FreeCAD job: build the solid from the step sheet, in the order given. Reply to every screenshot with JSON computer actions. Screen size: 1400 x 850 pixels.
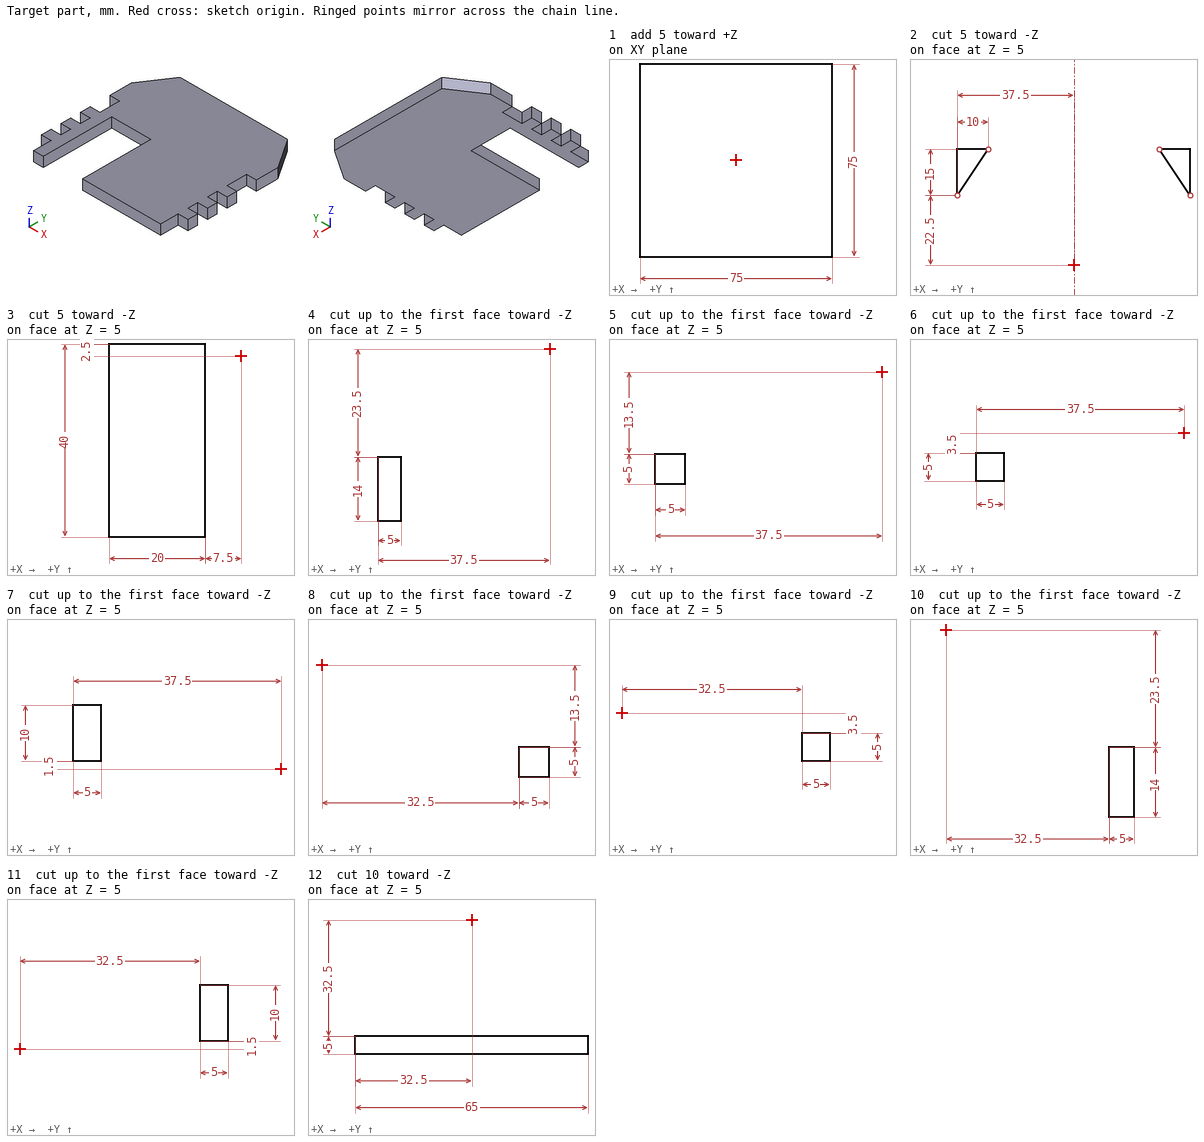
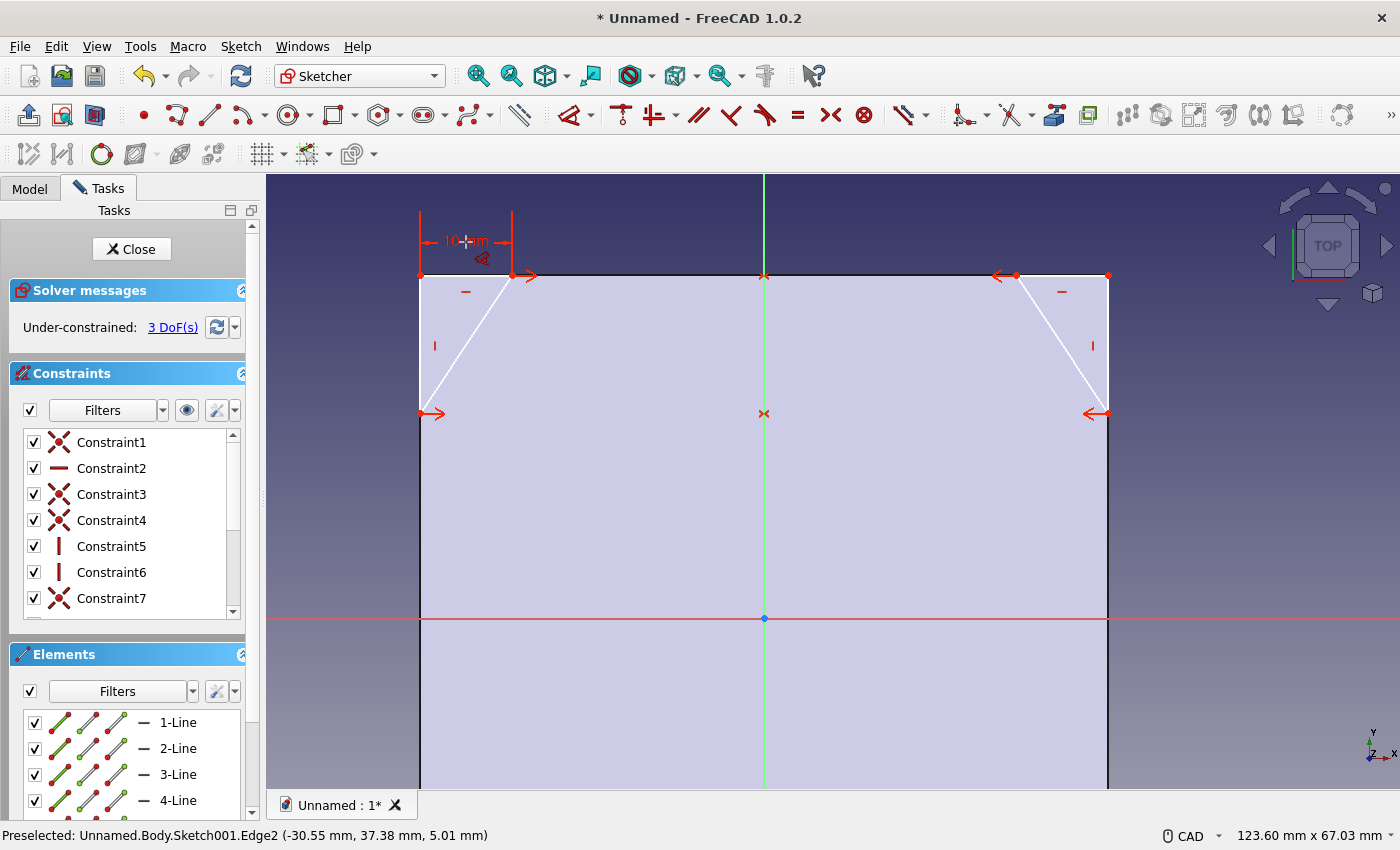
{"action": "left_click", "coordinate": [420, 317]}
{"action": "left_click", "coordinate": [386, 345]}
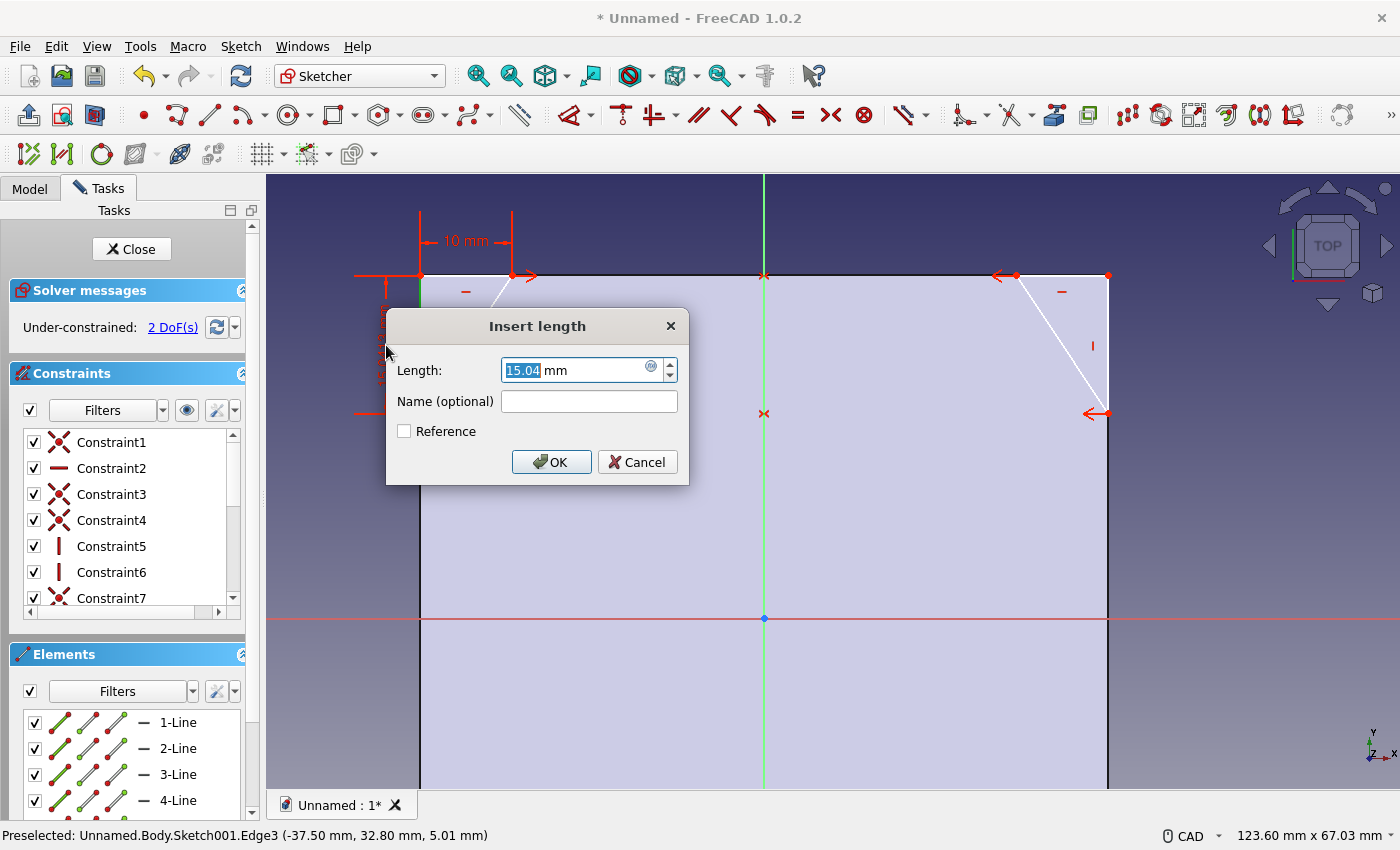
{"action": "type", "text": "15"}
{"action": "key", "text": "Return"}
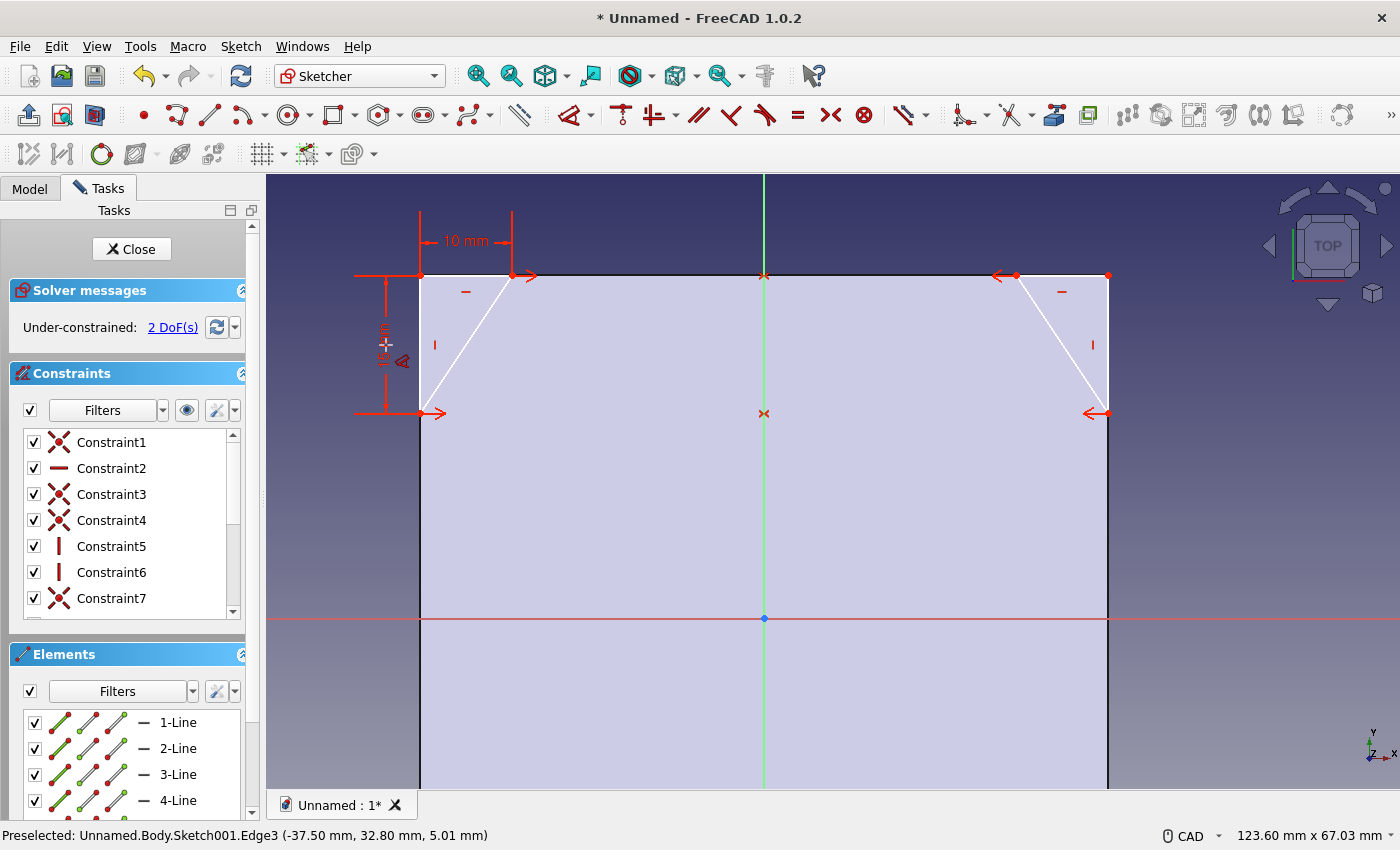
{"action": "left_click", "coordinate": [420, 414]}
{"action": "left_click", "coordinate": [592, 653]}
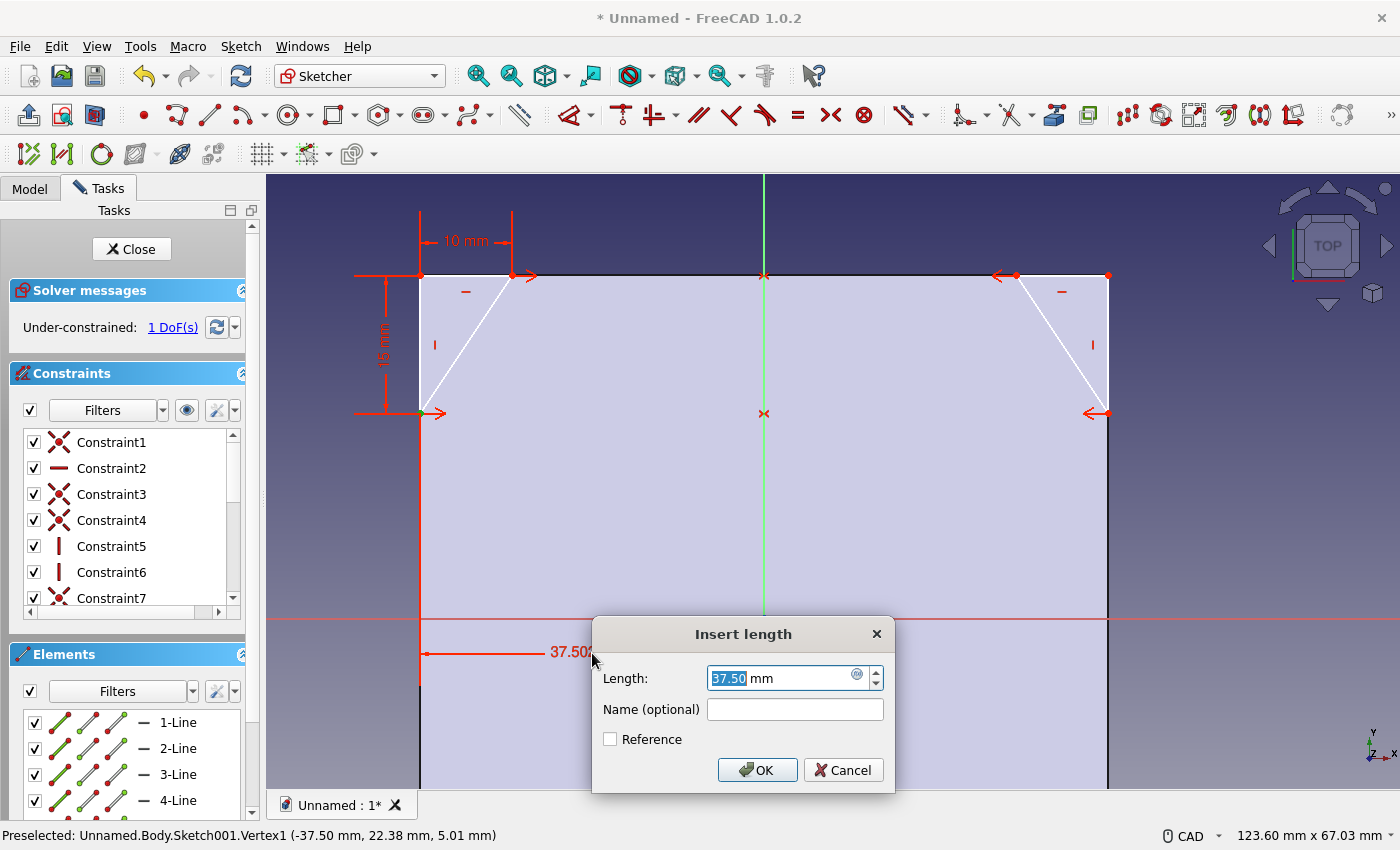
{"action": "type", "text": "37.5"}
{"action": "key", "text": "Return"}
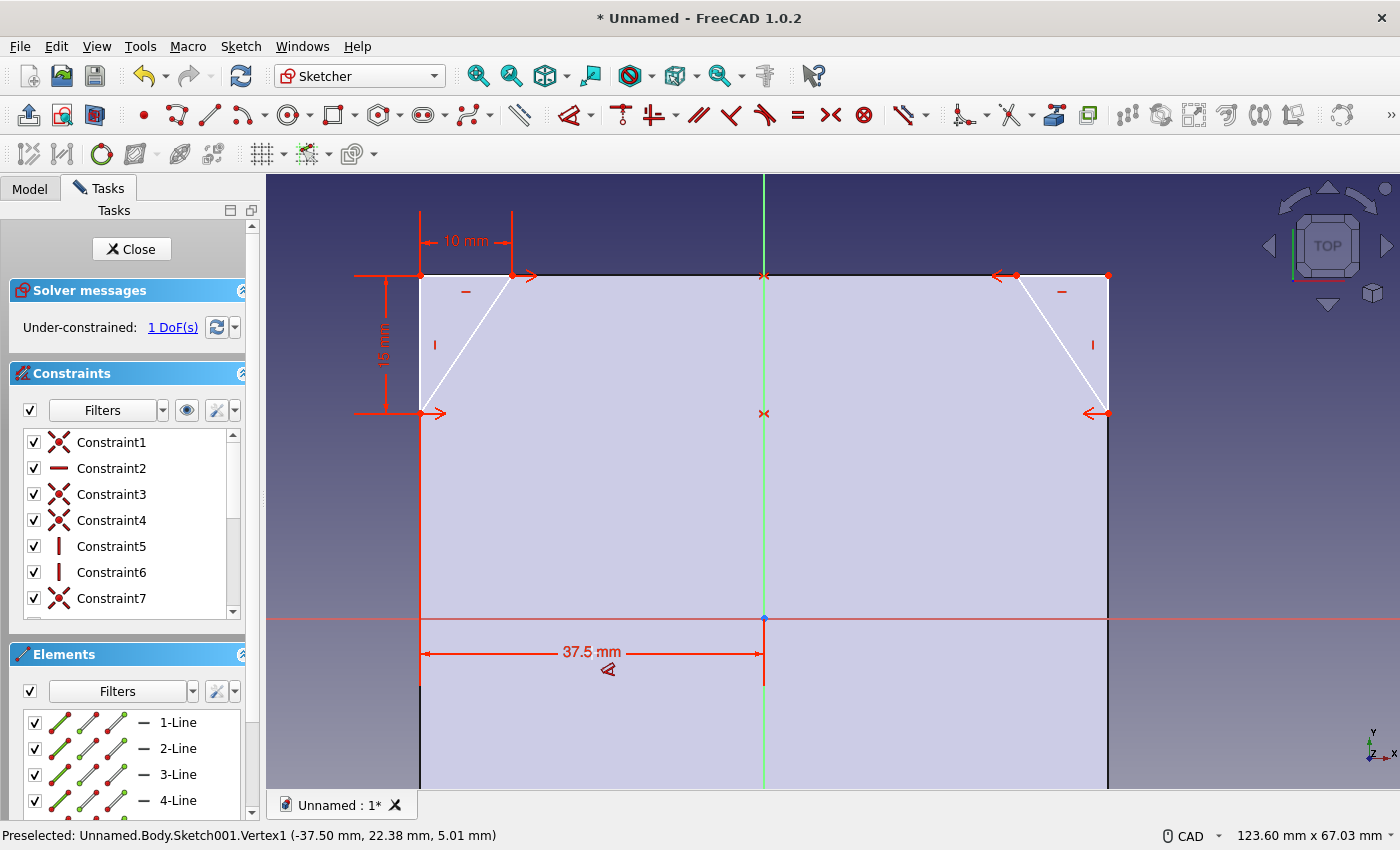
{"action": "left_click", "coordinate": [420, 414]}
{"action": "left_click", "coordinate": [386, 516]}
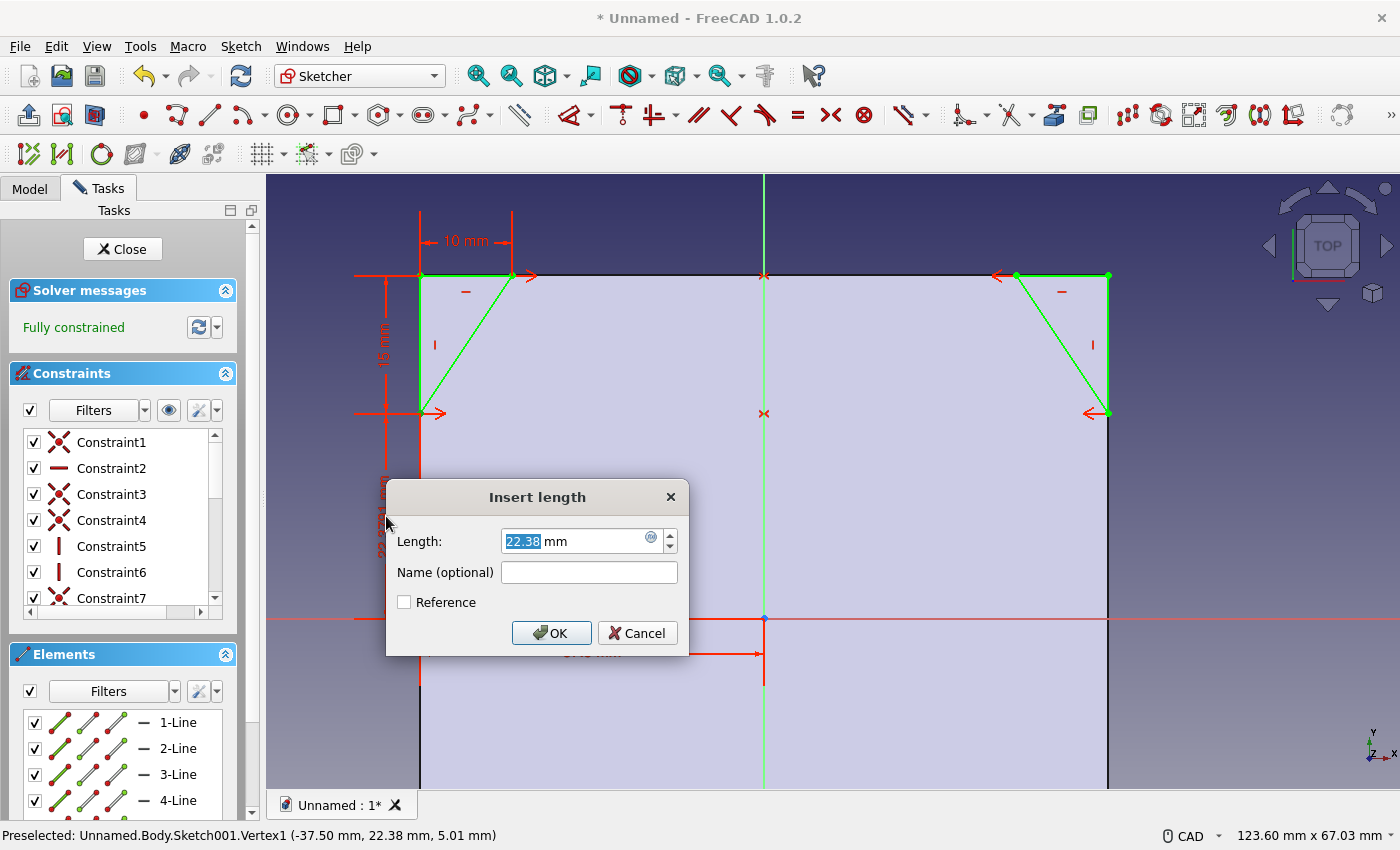
{"action": "type", "text": "22.5"}
{"action": "key", "text": "Return"}
{"action": "key", "text": "Escape"}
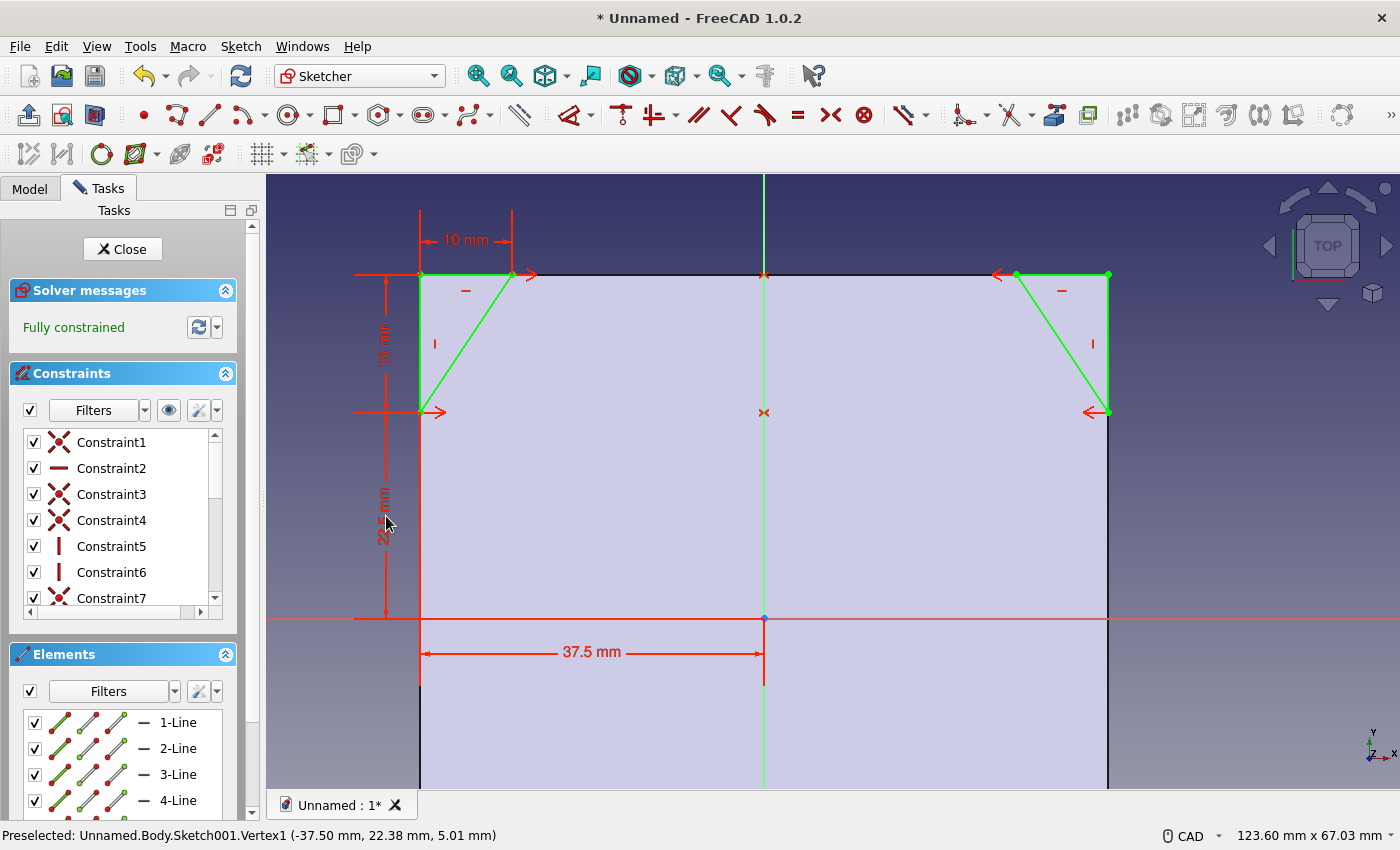
{"action": "left_click", "coordinate": [123, 249]}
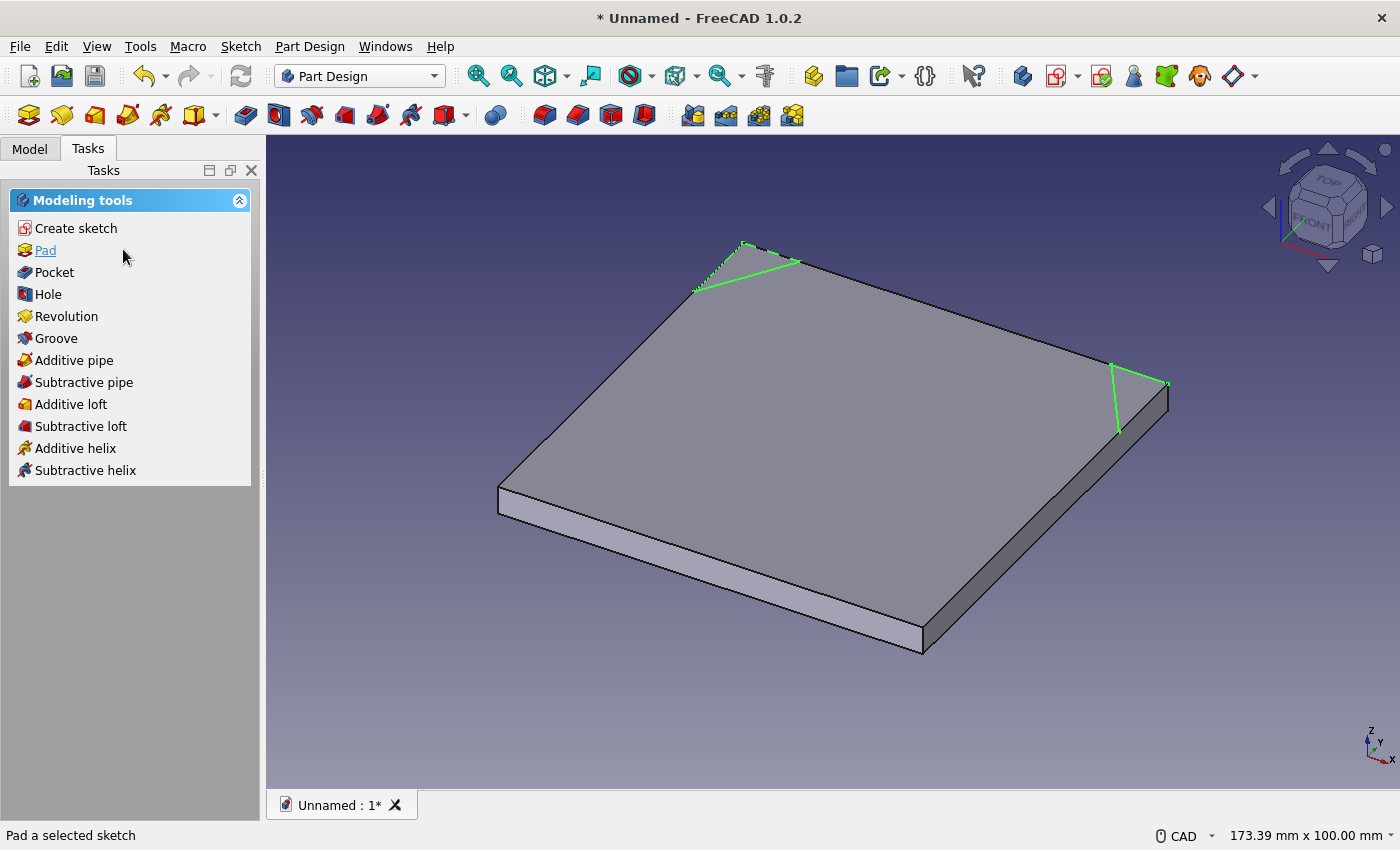
{"action": "left_click", "coordinate": [246, 116]}